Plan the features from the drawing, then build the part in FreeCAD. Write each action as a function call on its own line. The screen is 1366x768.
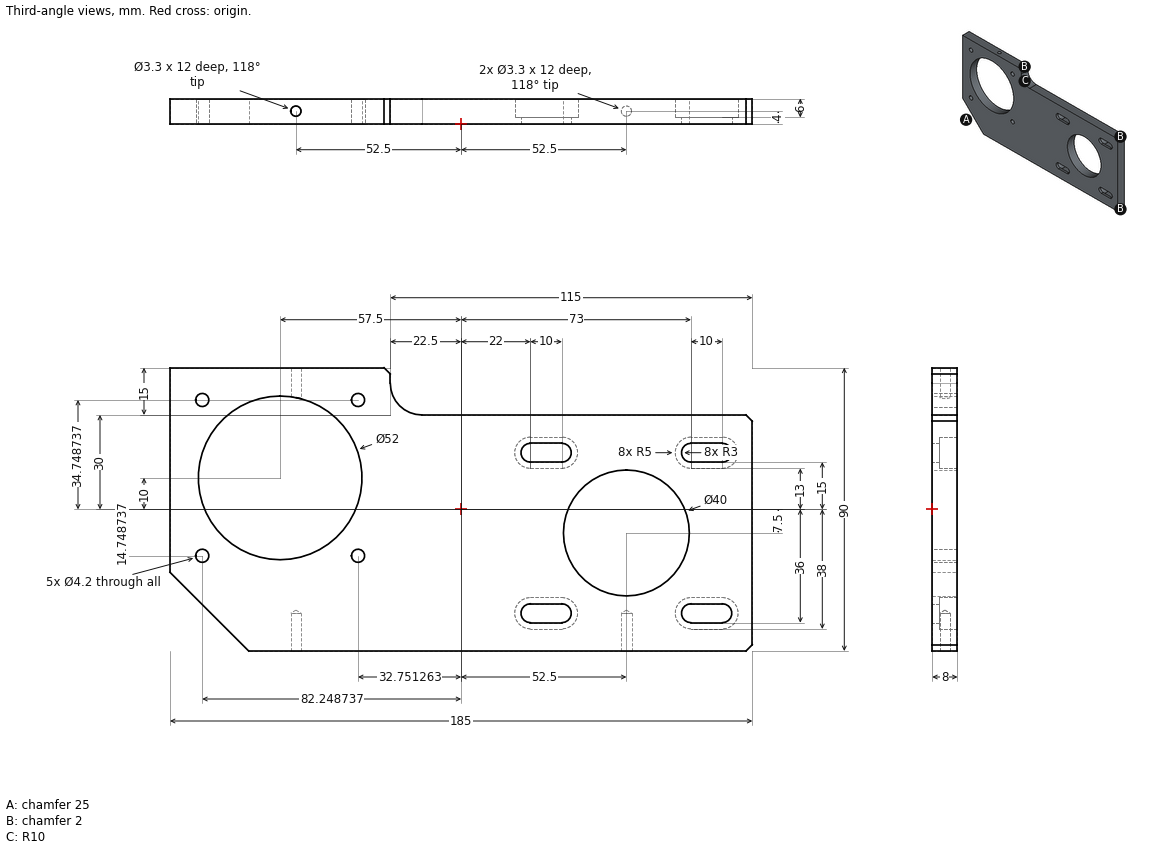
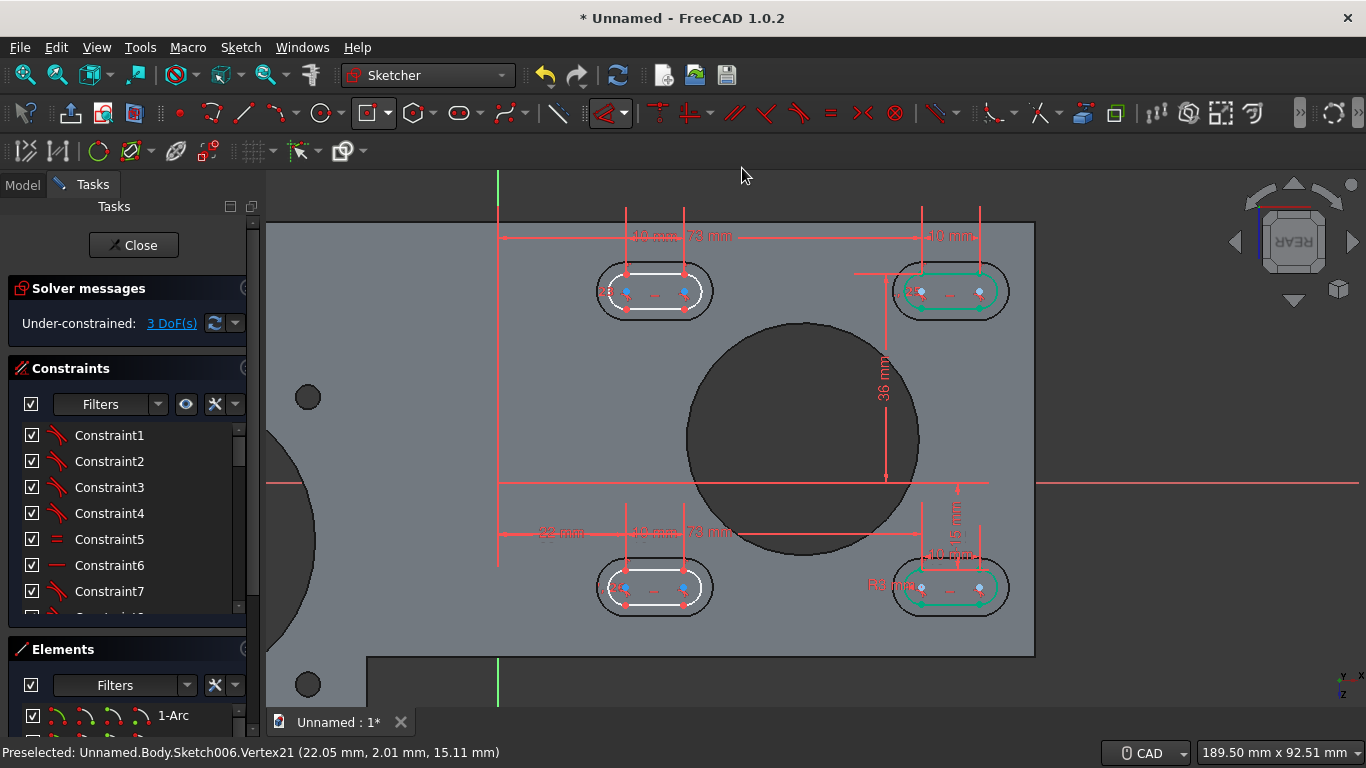
click(626, 570)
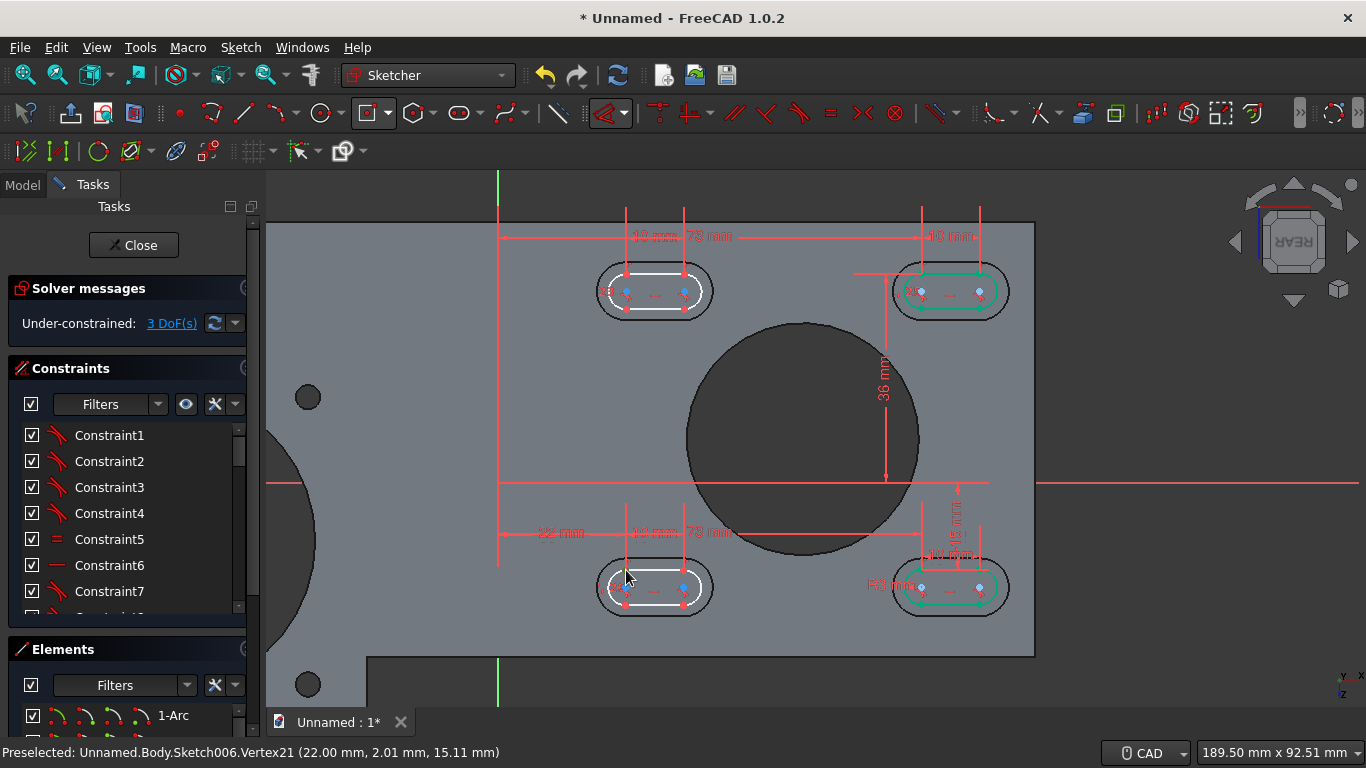
key(i)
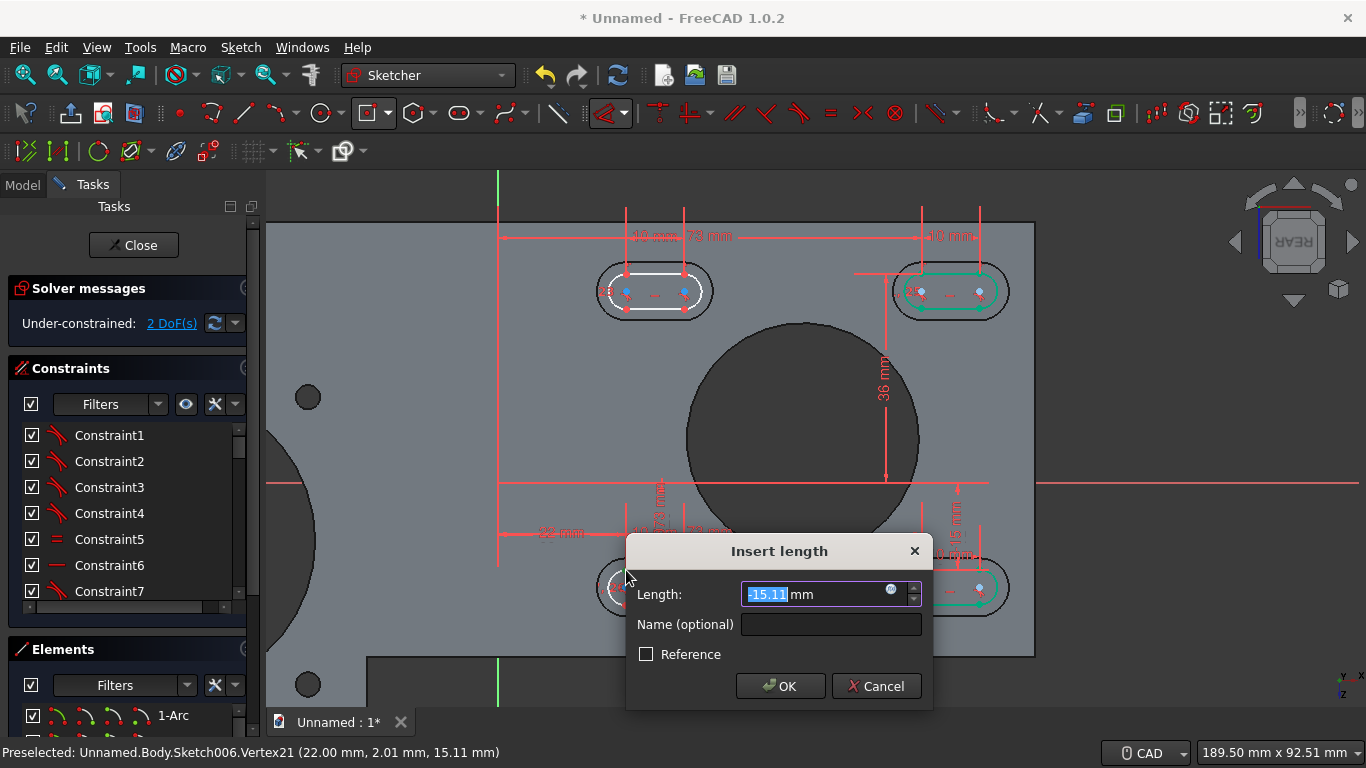
text(-15)
key(Return)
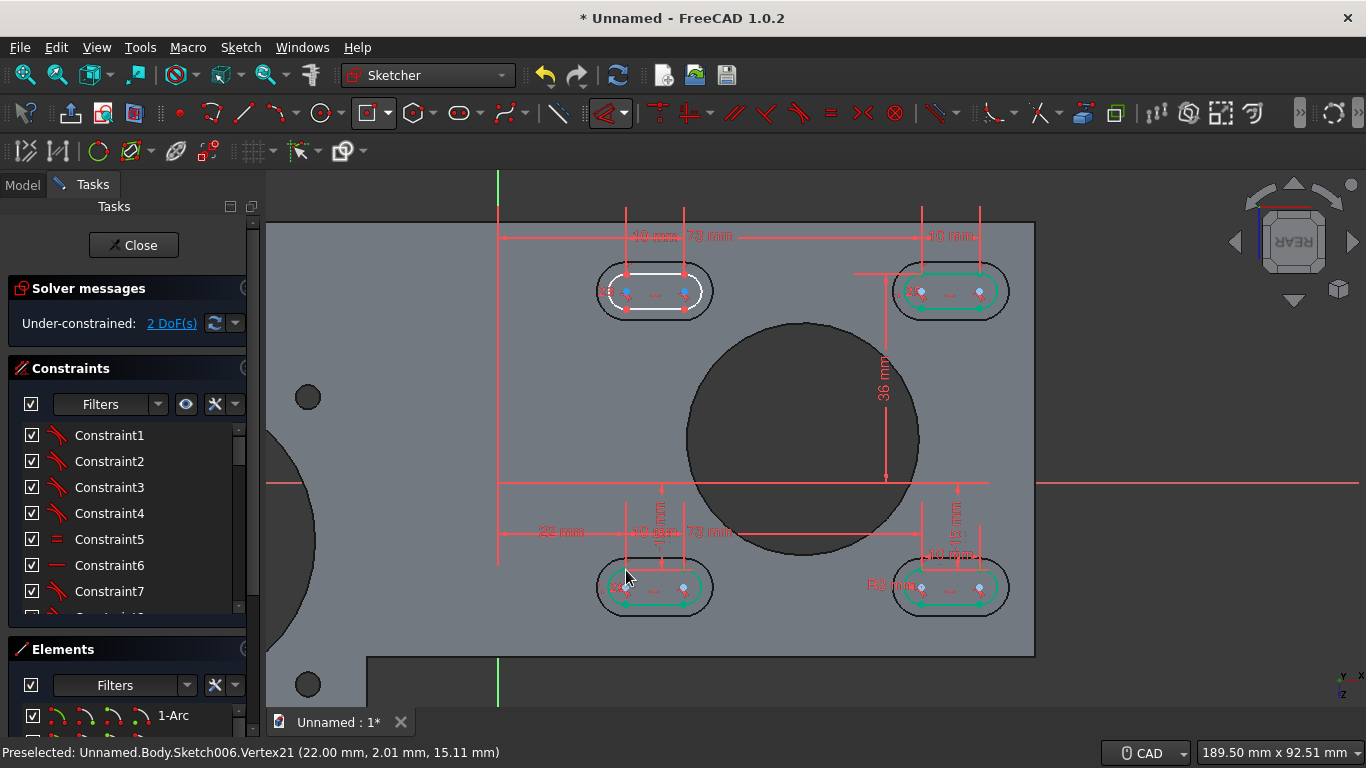
click(626, 274)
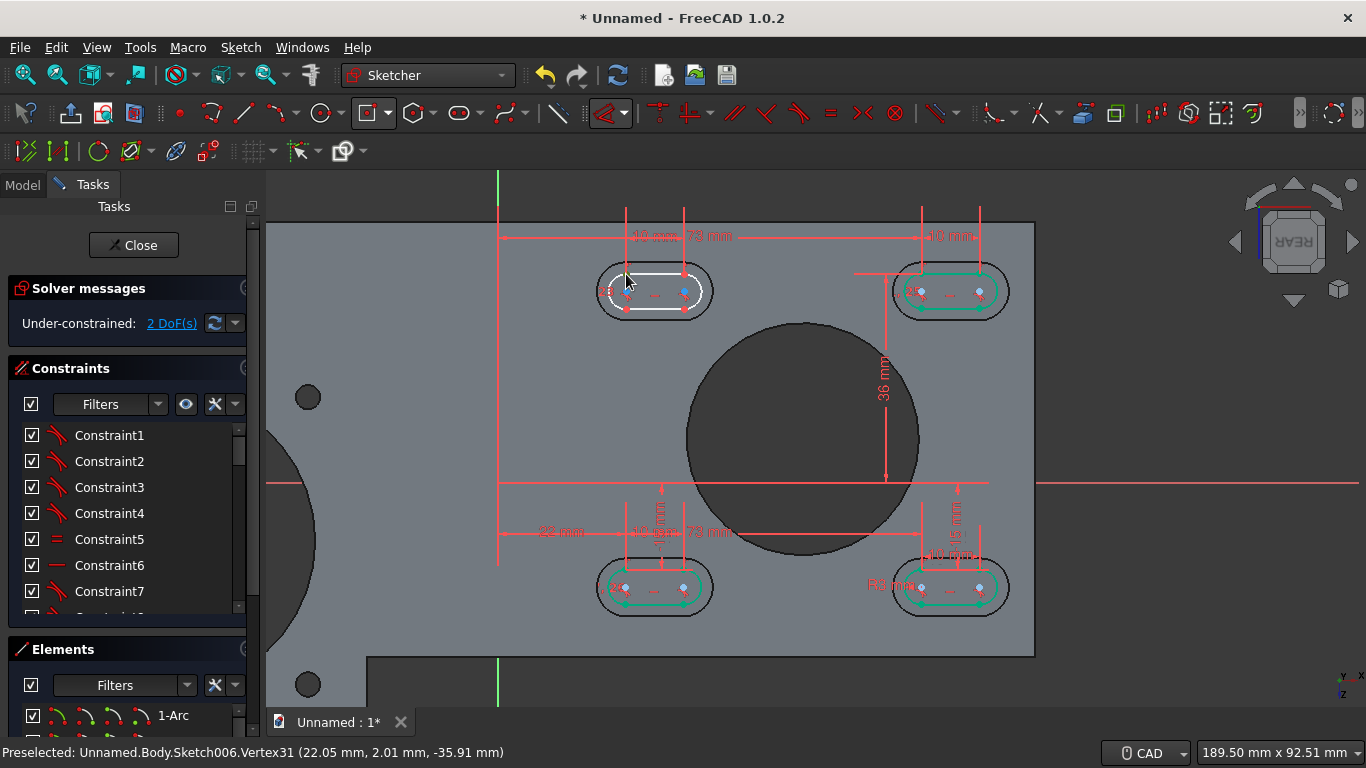
click(626, 114)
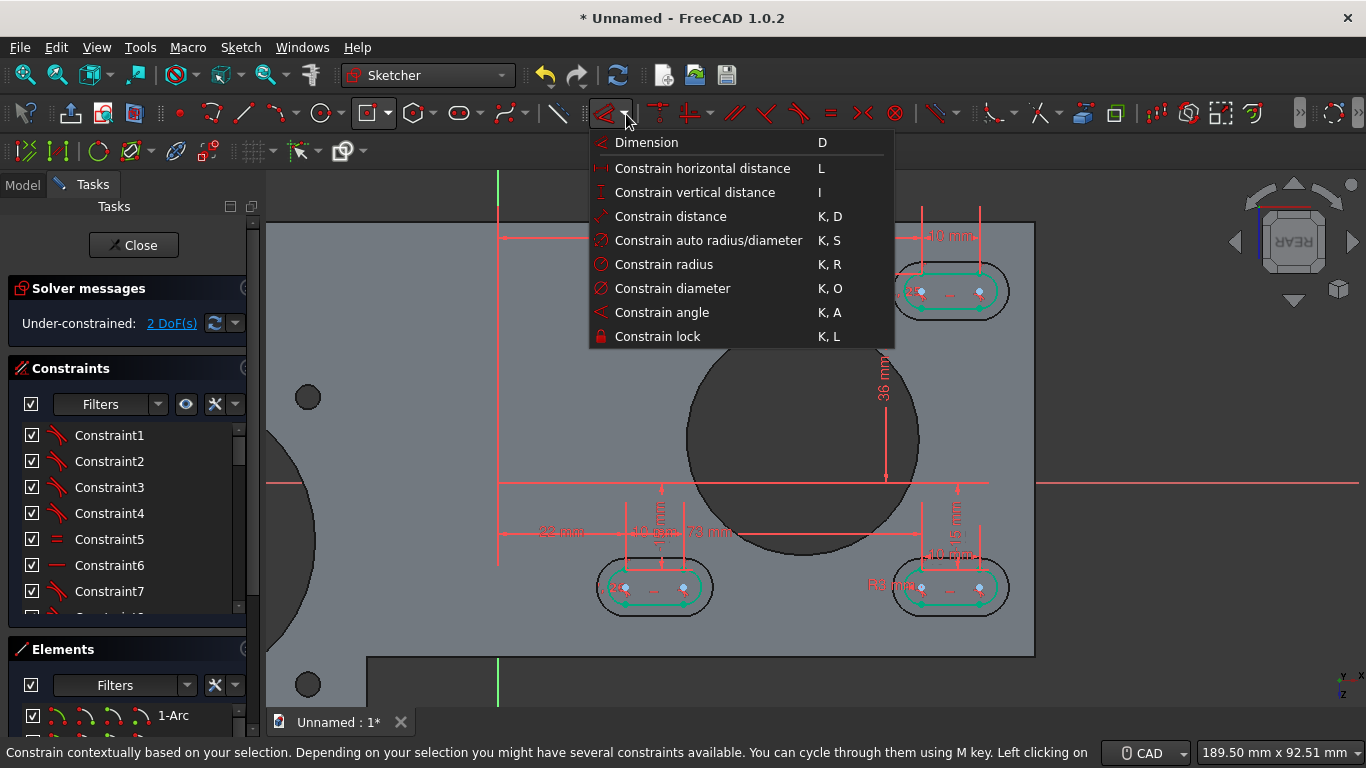
click(742, 168)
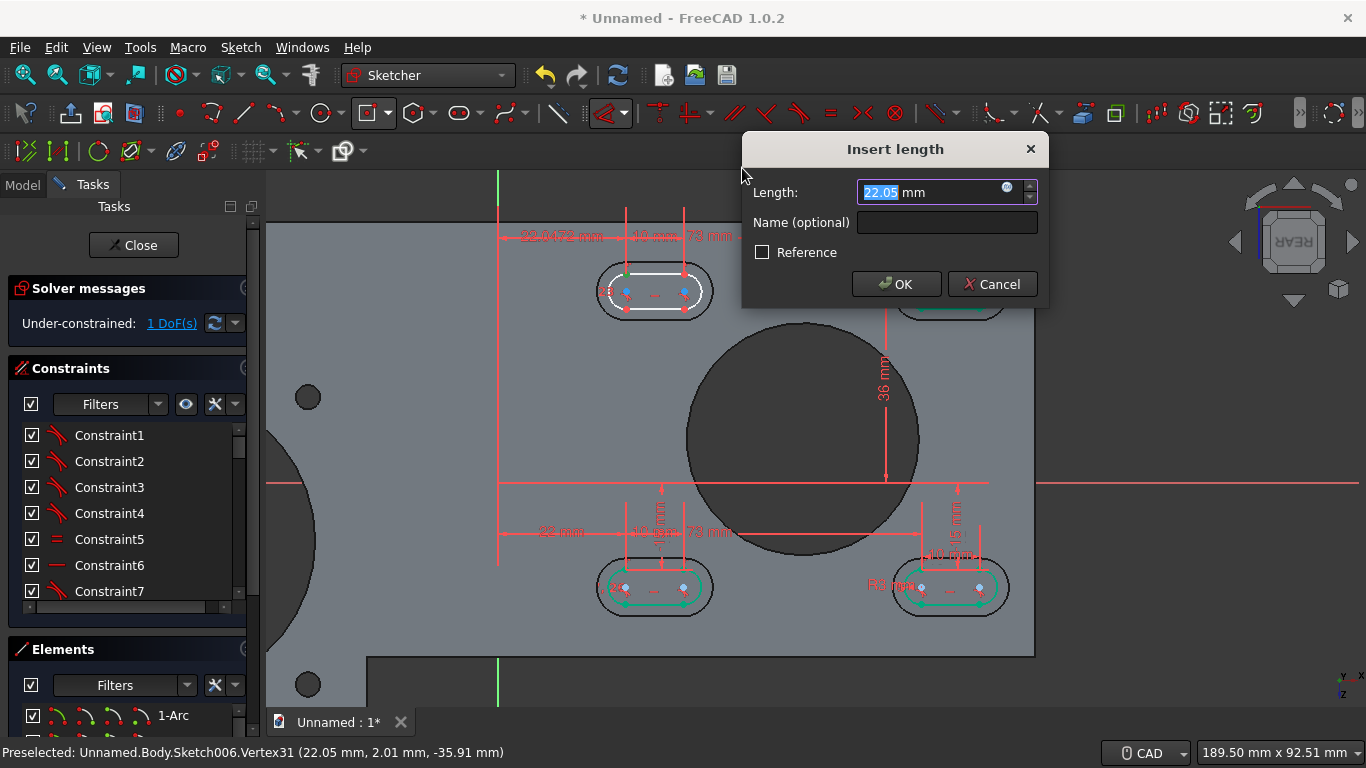
text(22)
key(Return)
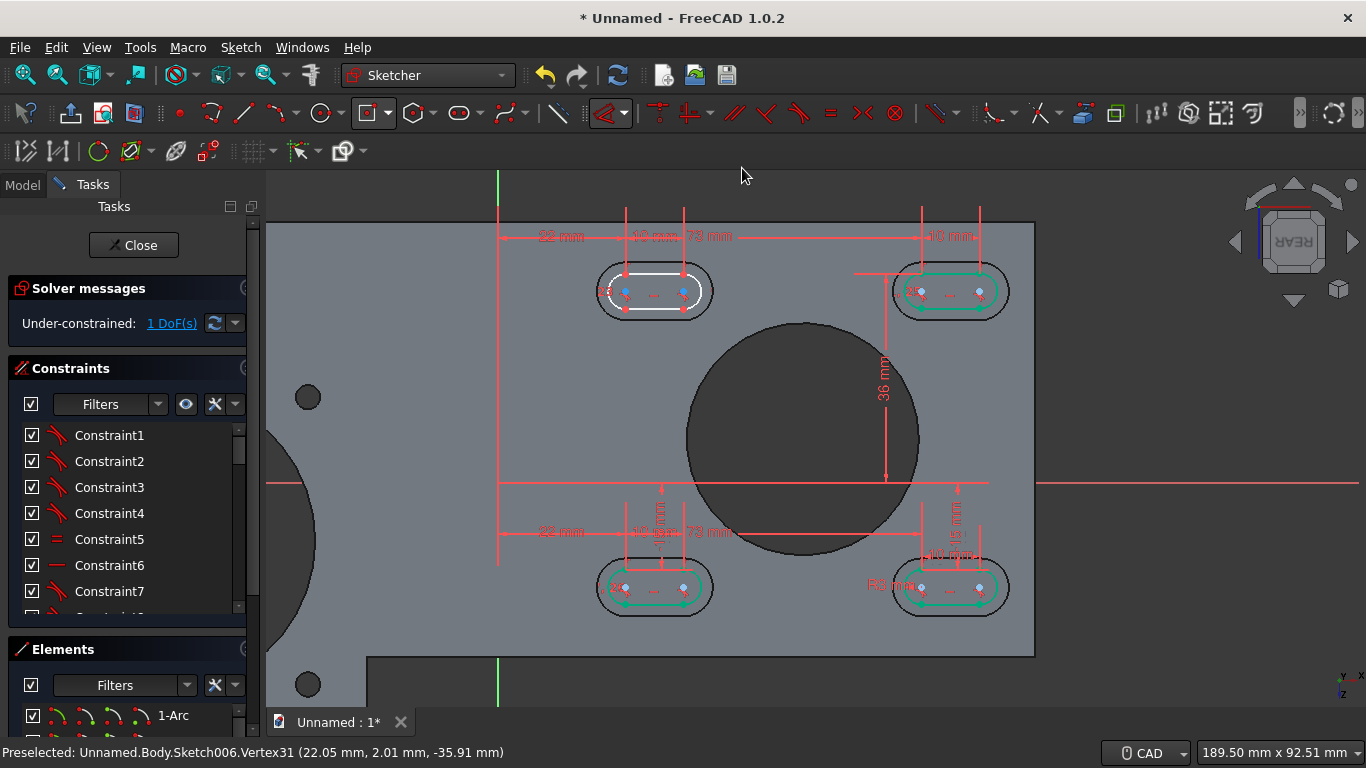
click(626, 274)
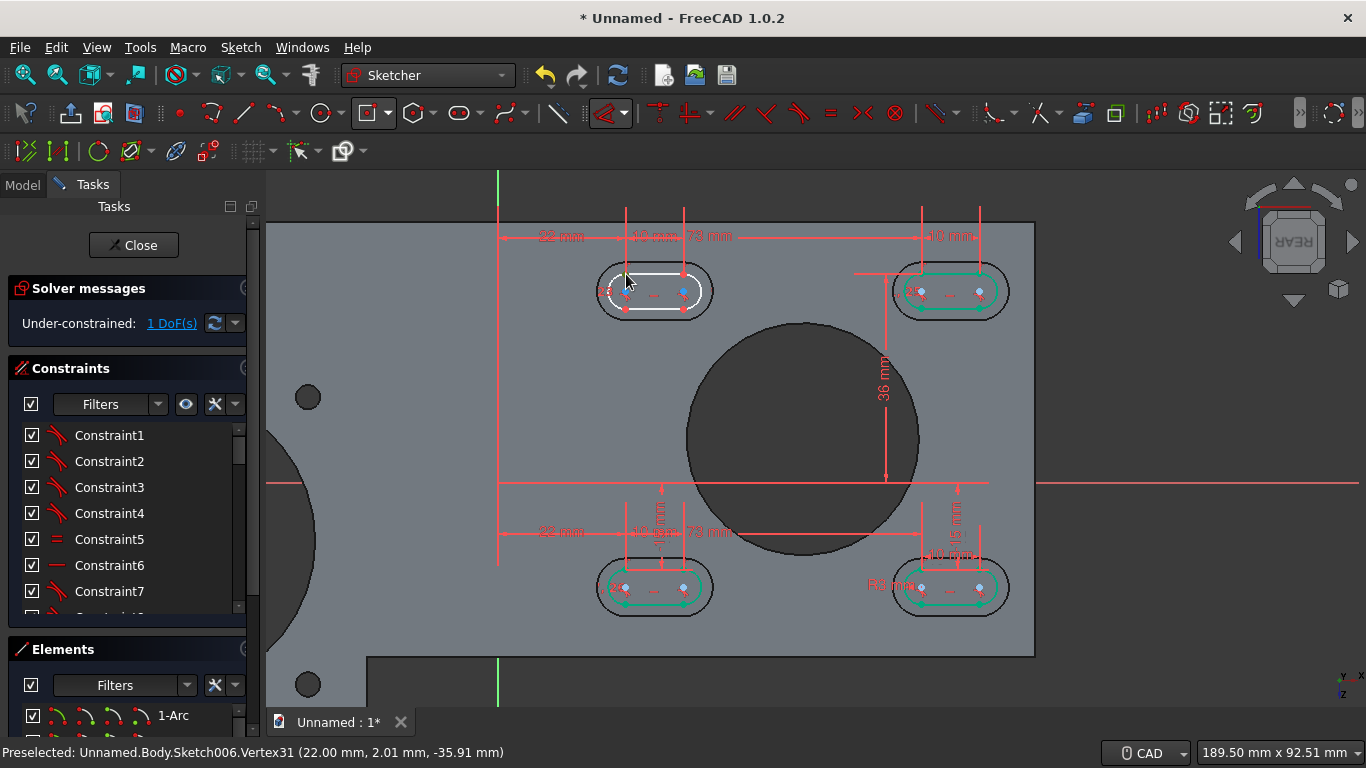
key(i)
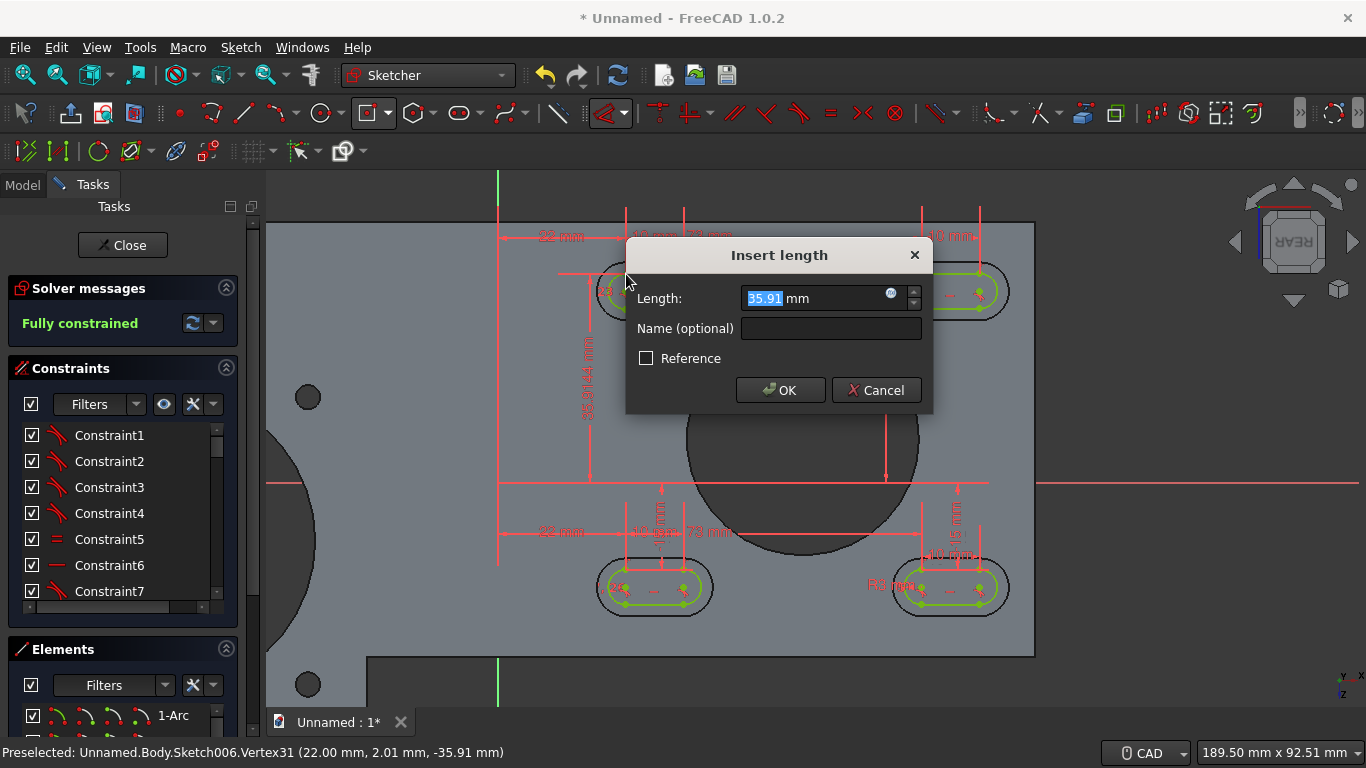
text(36)
key(Return)